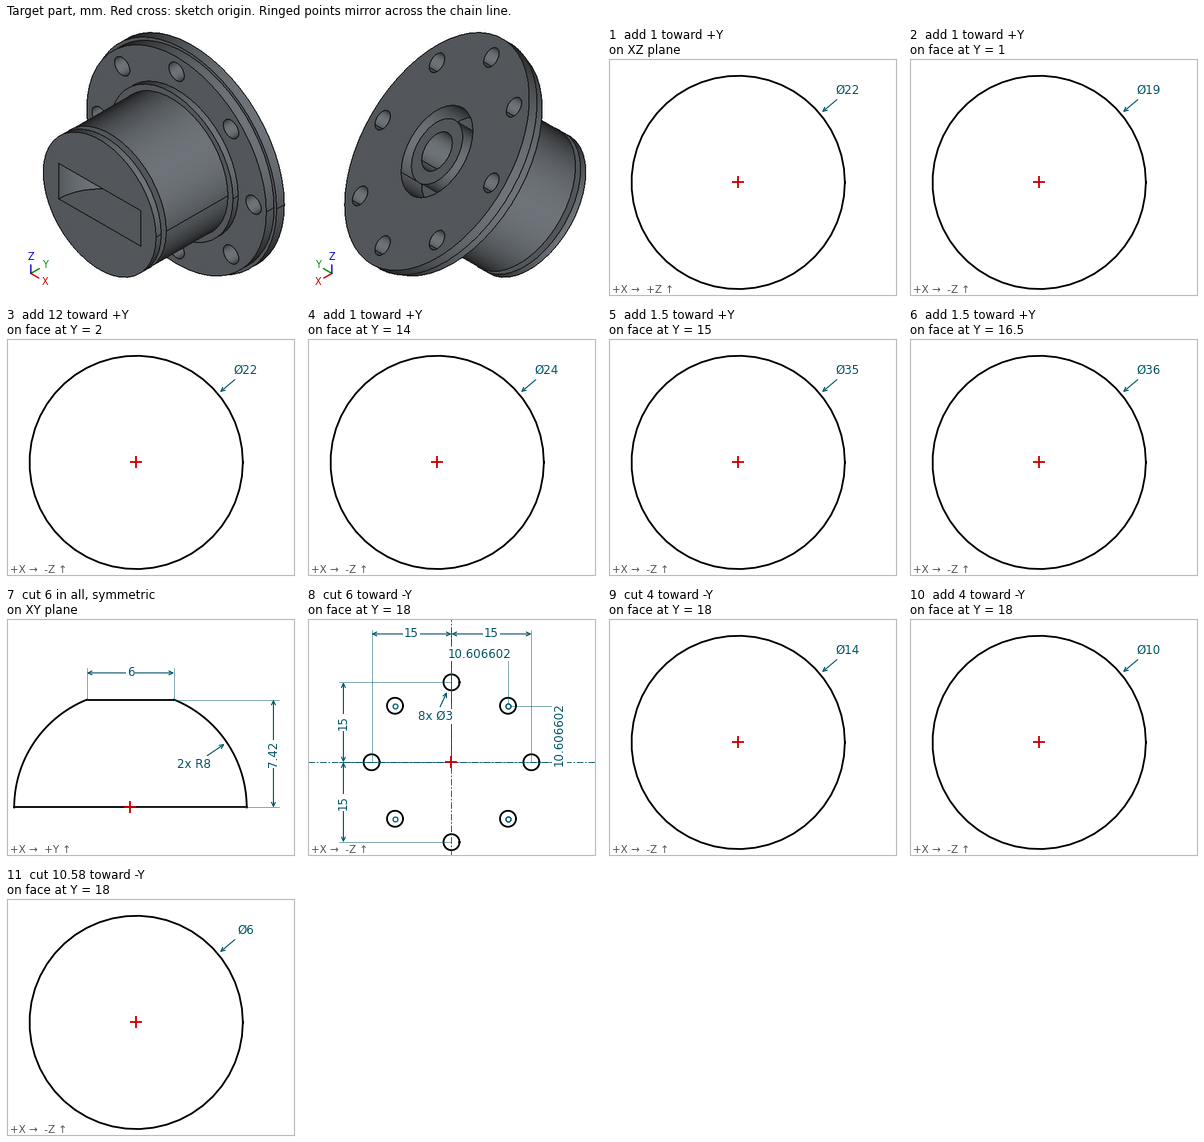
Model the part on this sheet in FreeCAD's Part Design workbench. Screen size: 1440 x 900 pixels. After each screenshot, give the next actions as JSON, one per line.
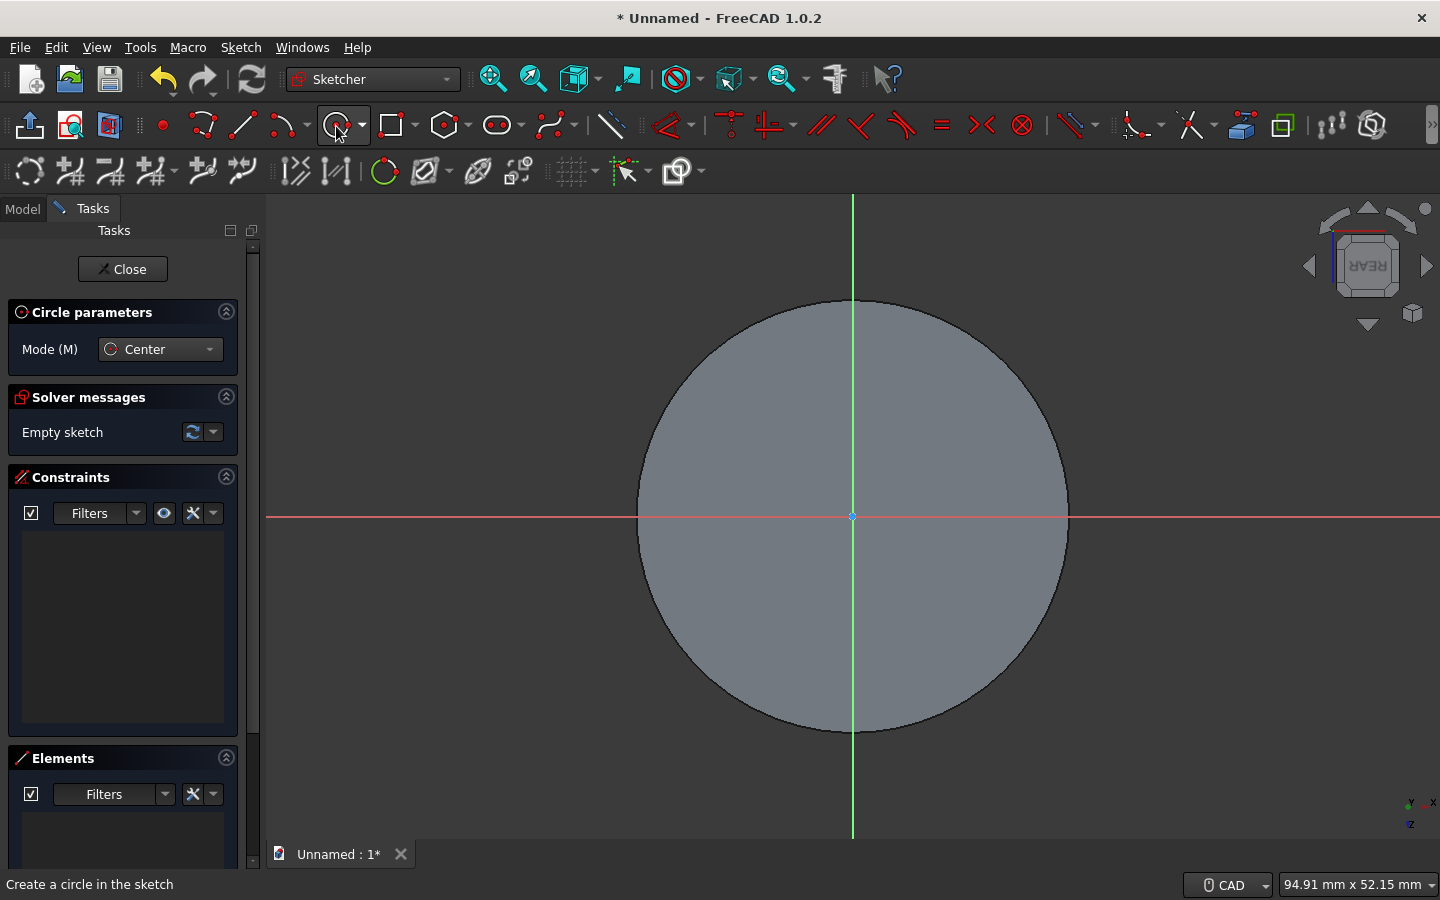
{"action": "left_click", "coordinate": [853, 516]}
{"action": "mouse_move", "coordinate": [1010, 359]}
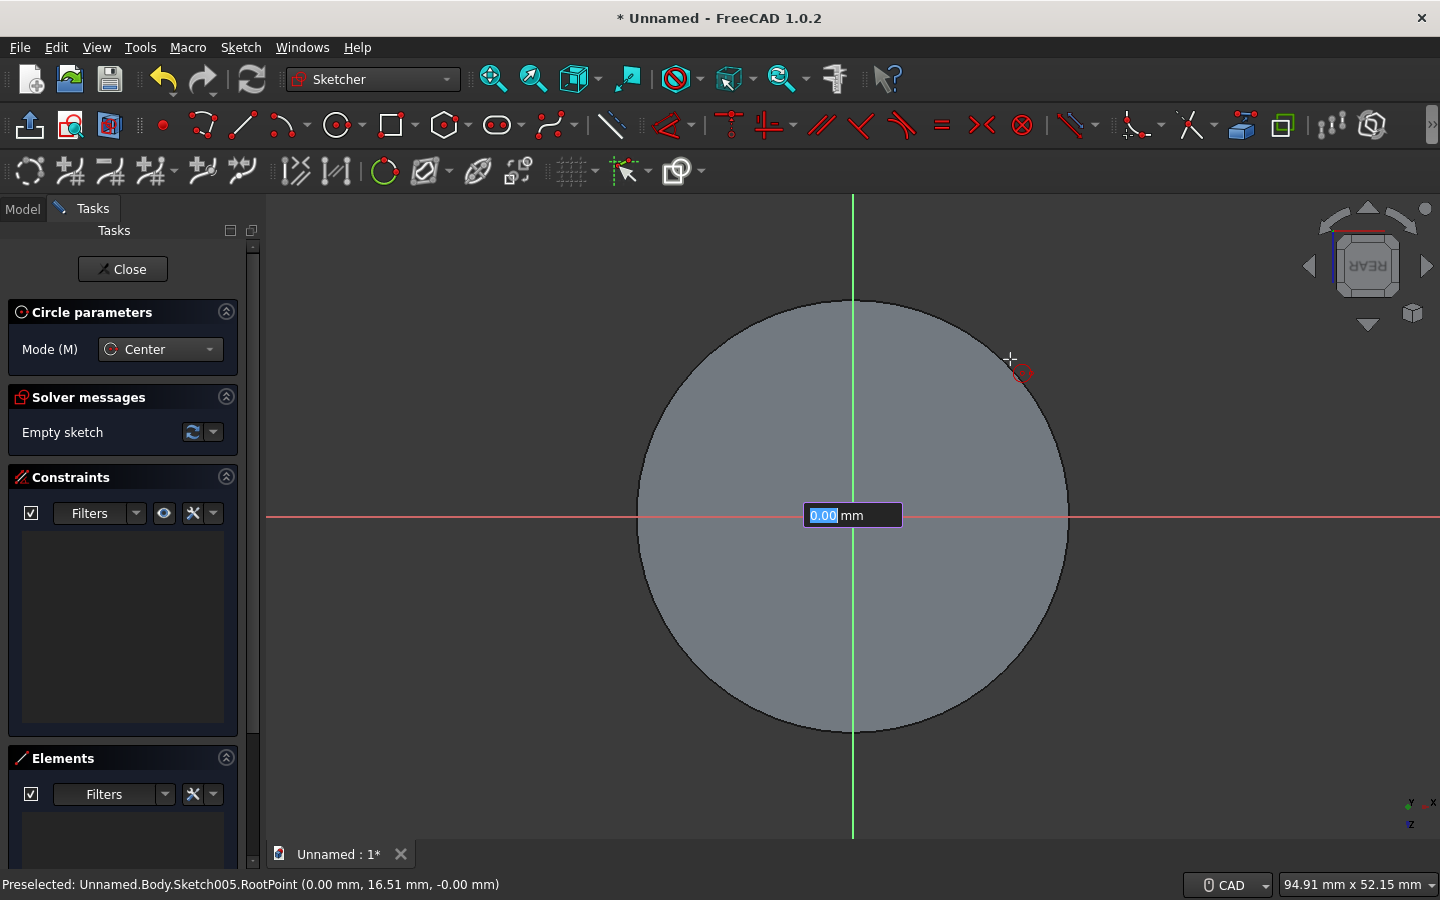
{"action": "type", "text": "36"}
{"action": "key", "text": "Return"}
{"action": "key", "text": "Escape"}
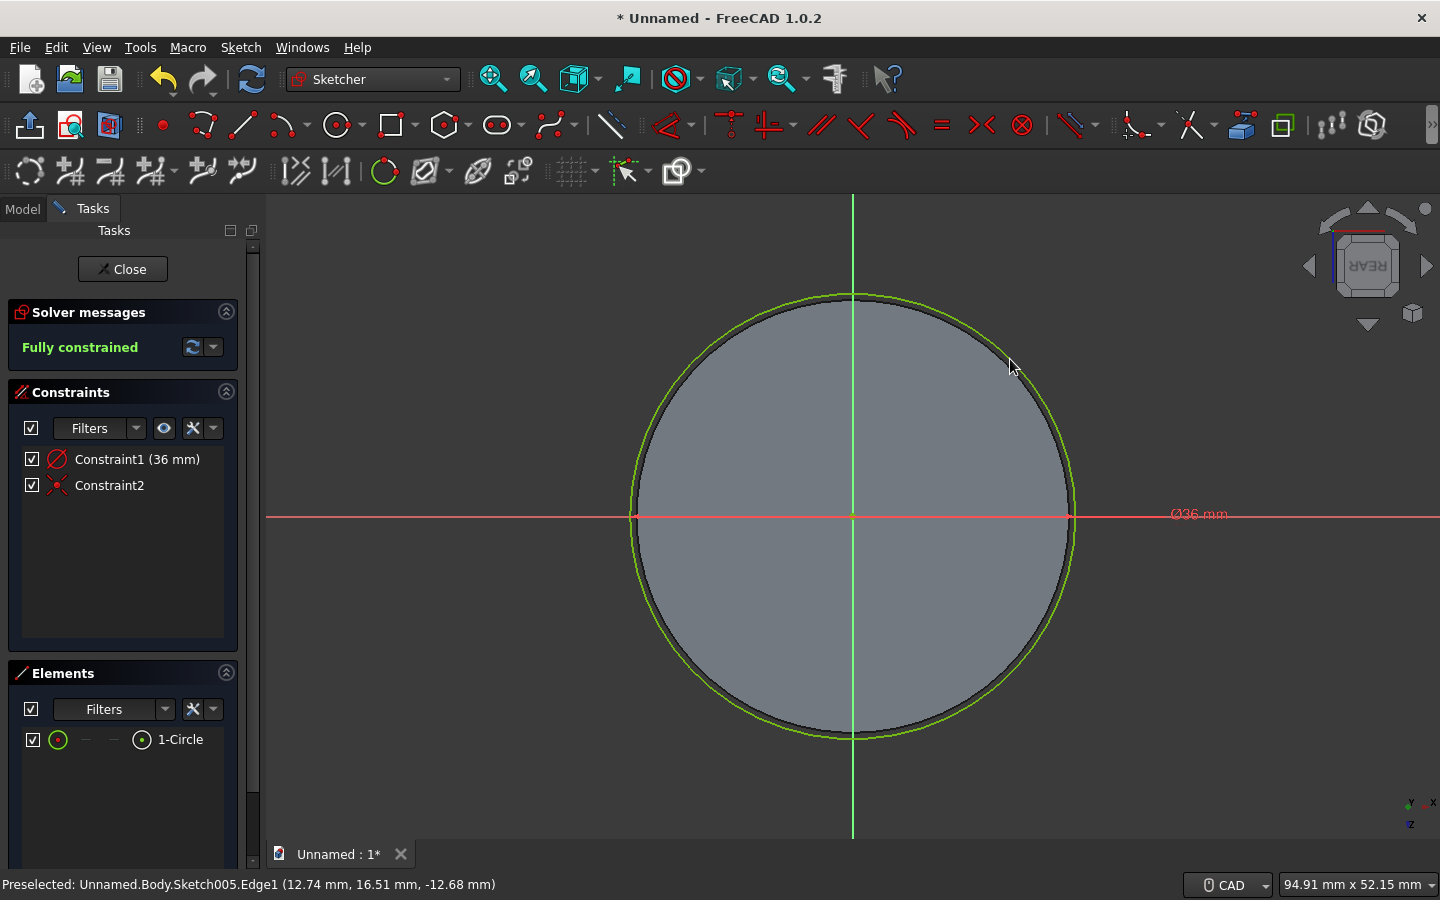
{"action": "left_click", "coordinate": [123, 269]}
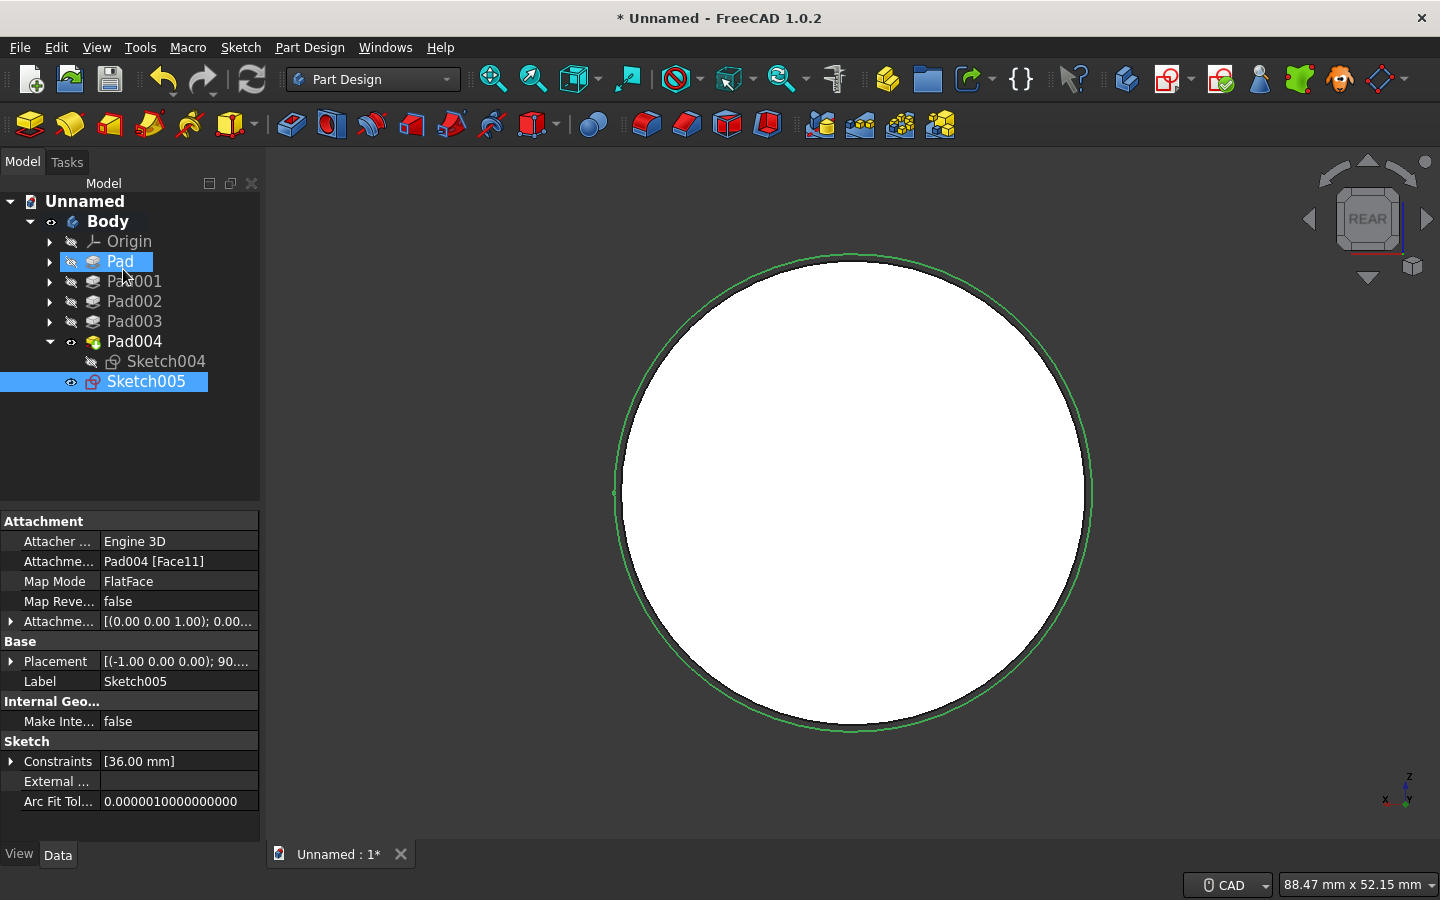
{"action": "left_click", "coordinate": [30, 124]}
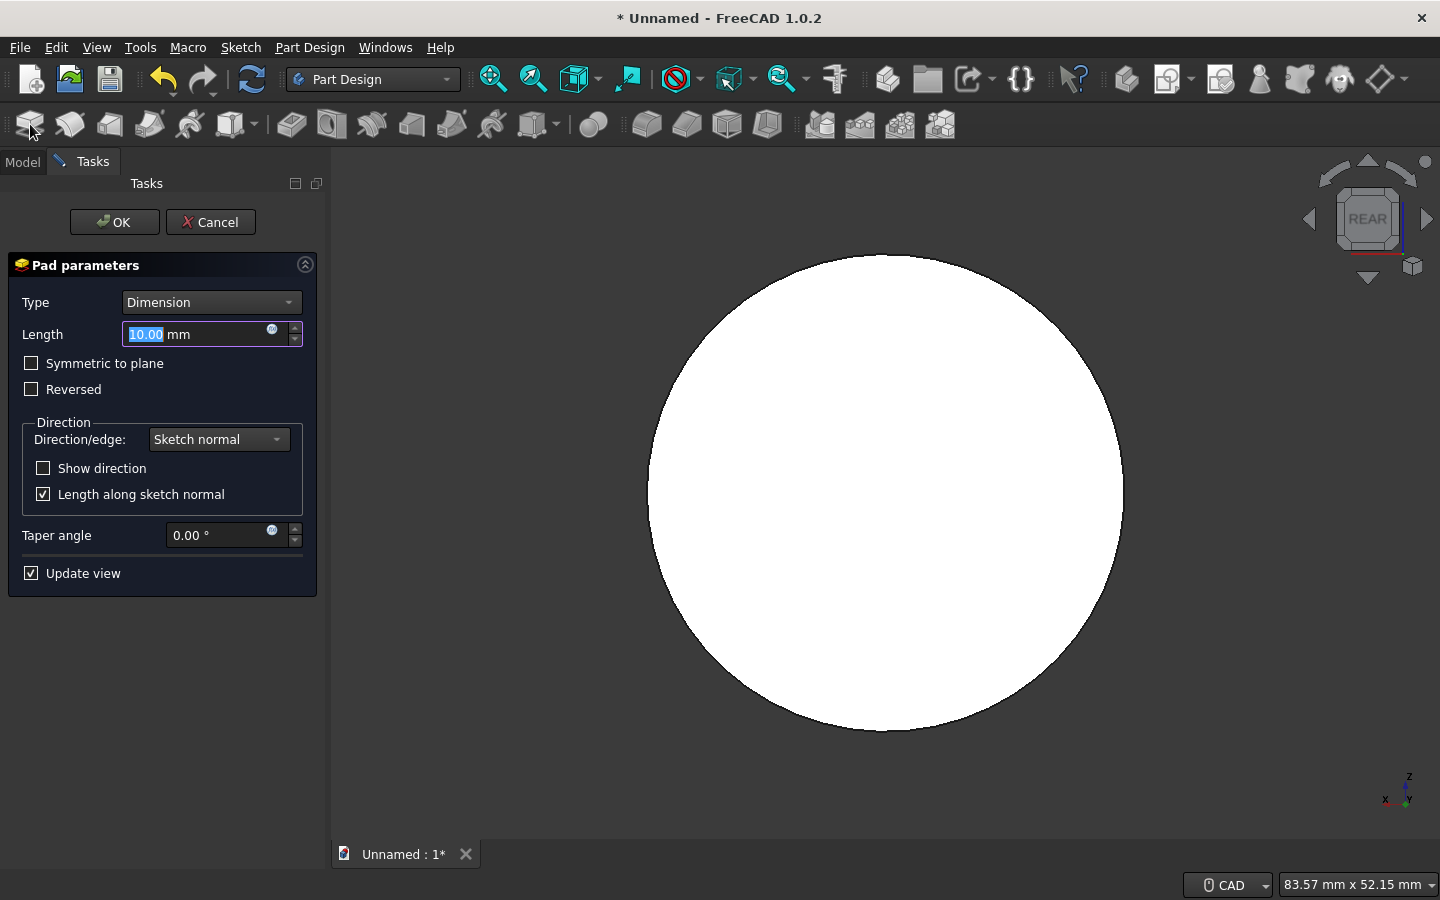
{"action": "type", "text": "1.5"}
{"action": "key", "text": "Tab"}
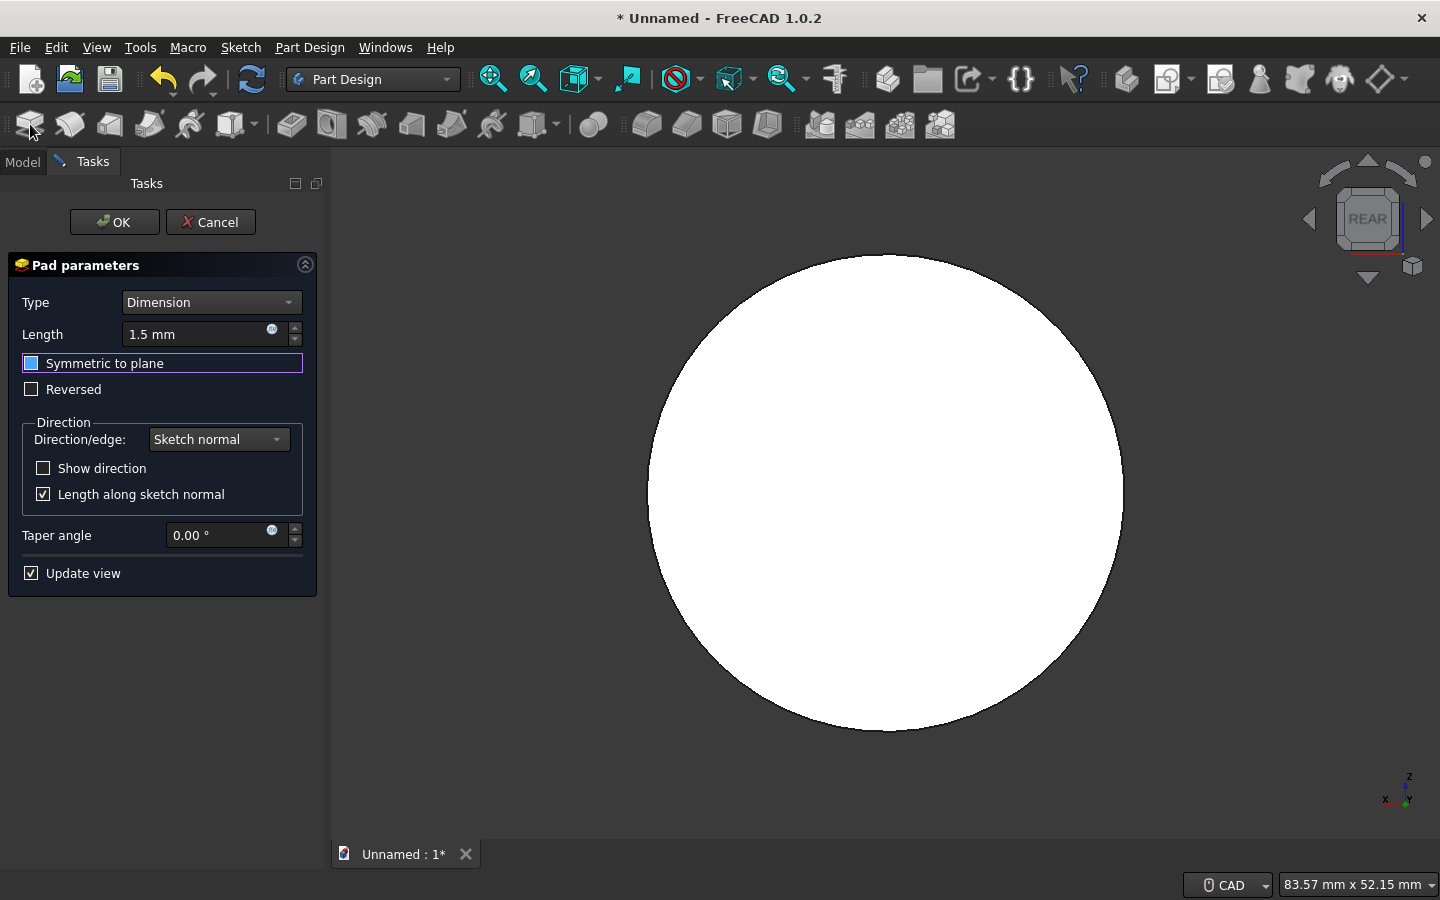
{"action": "left_click", "coordinate": [115, 222]}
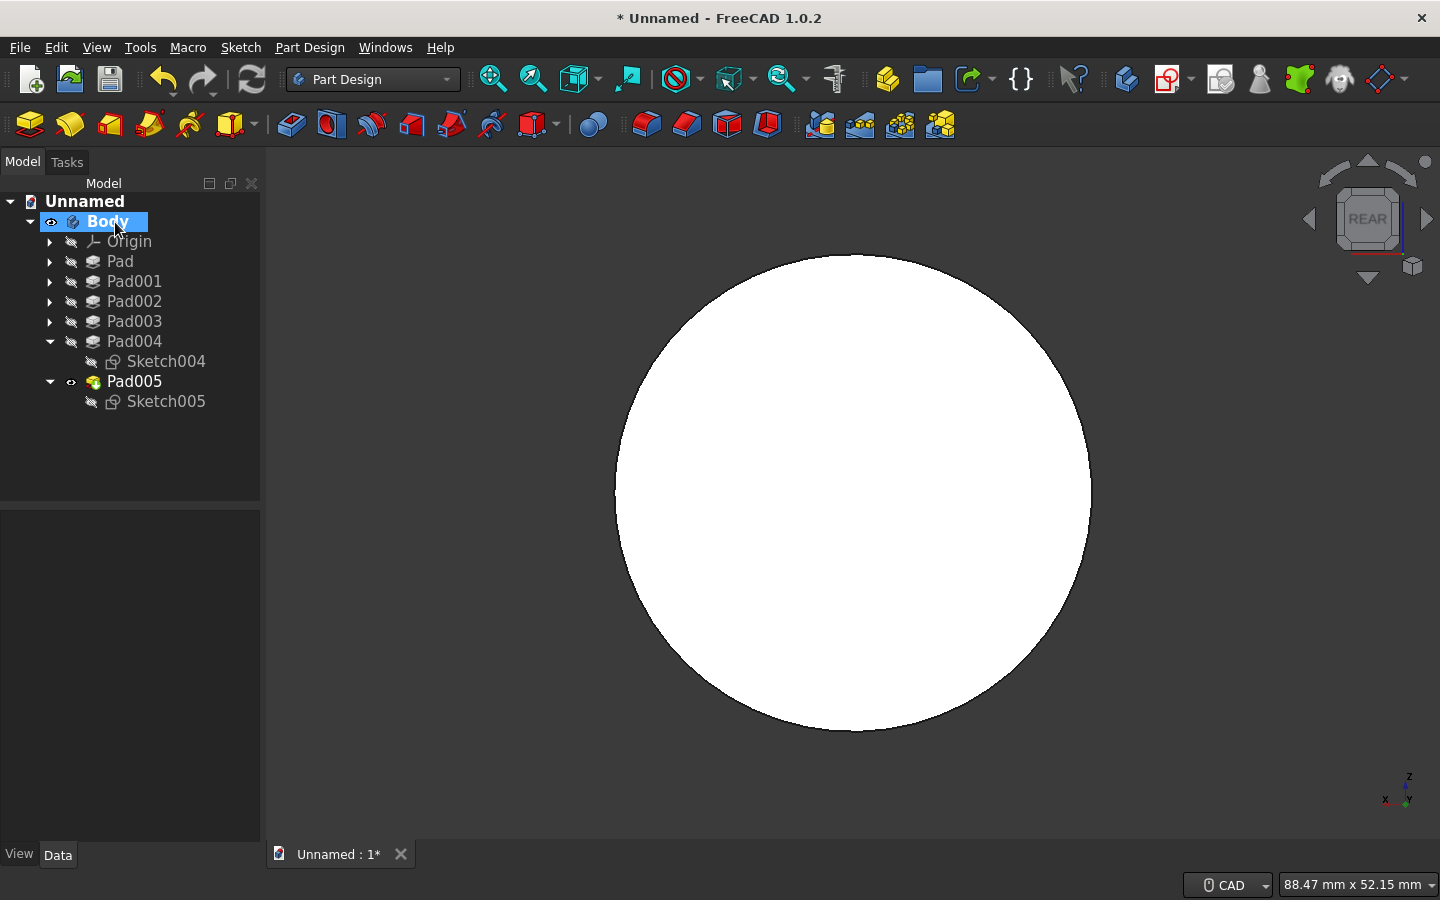
{"action": "left_click", "coordinate": [1168, 80]}